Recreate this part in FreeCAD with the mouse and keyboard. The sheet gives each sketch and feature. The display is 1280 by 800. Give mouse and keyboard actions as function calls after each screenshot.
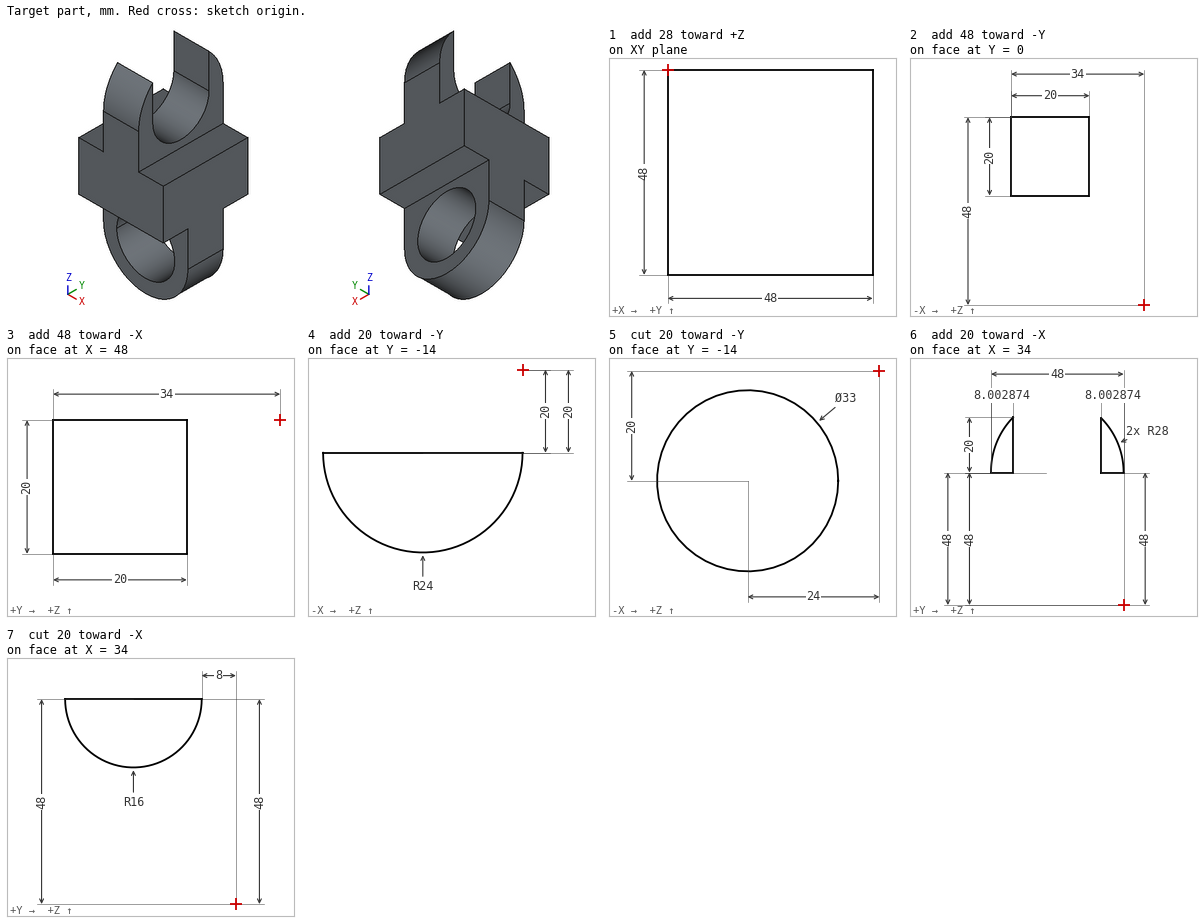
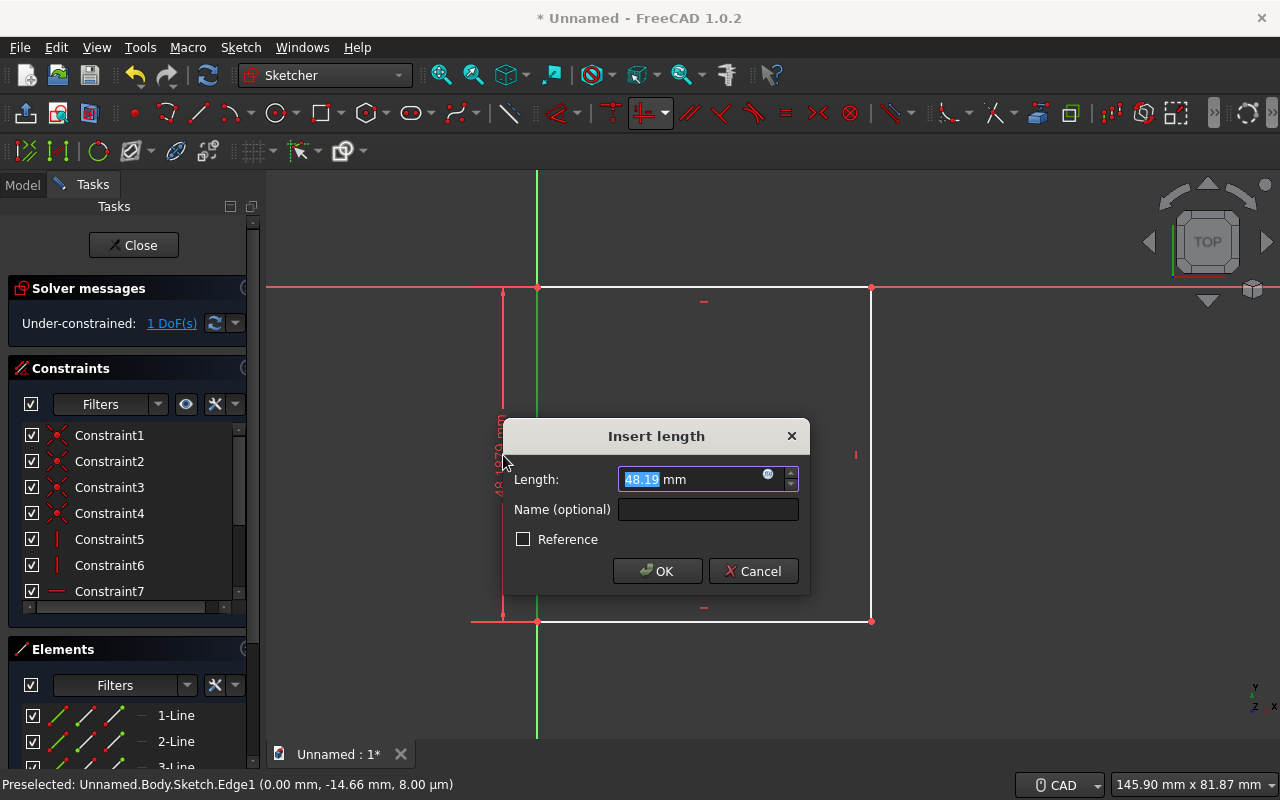
text(48)
key(Return)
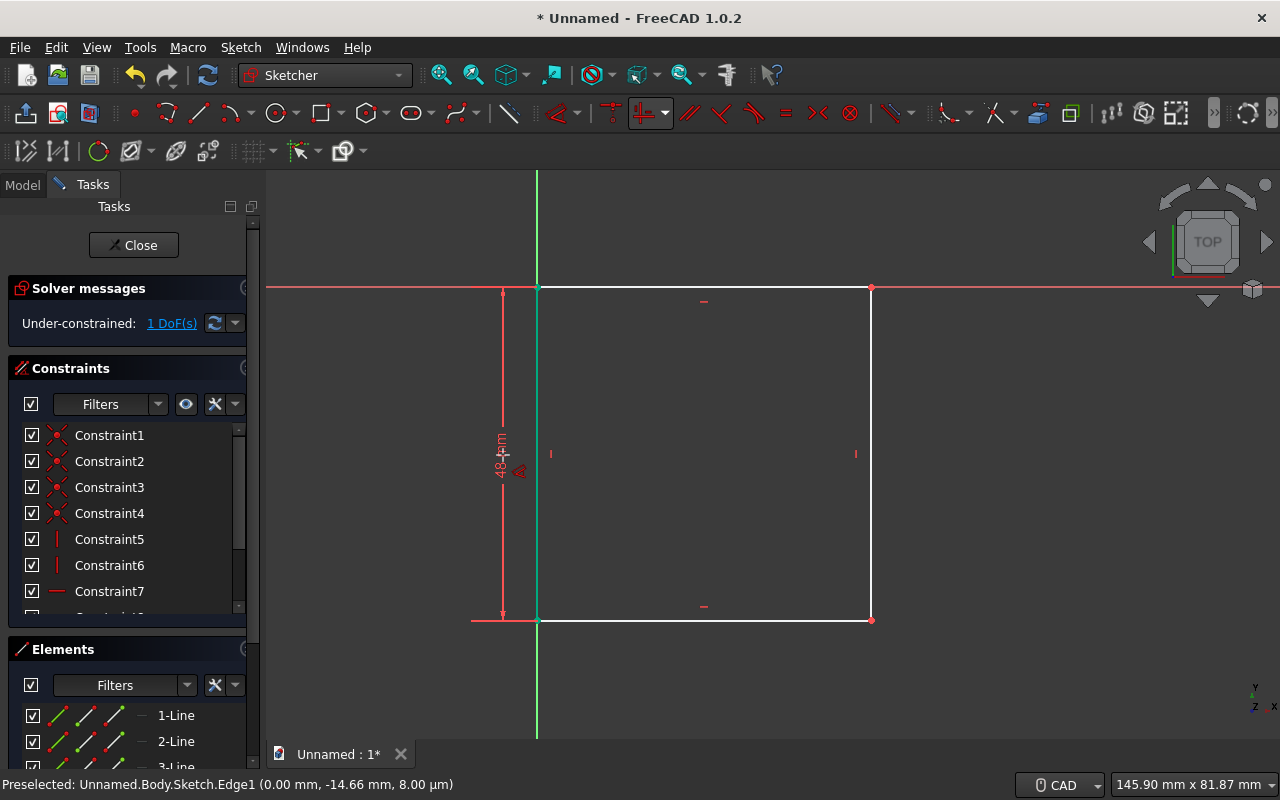
click(637, 621)
click(704, 655)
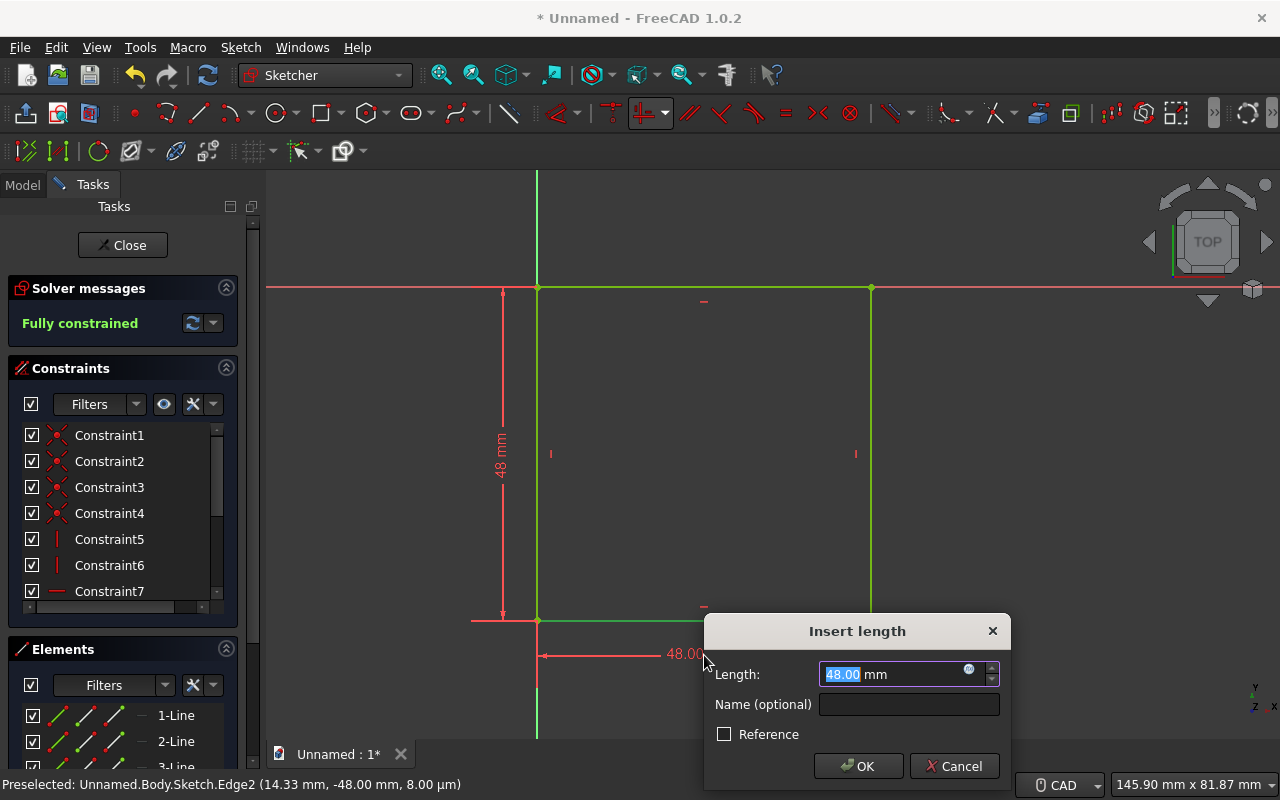
text(48)
key(Return)
key(Escape)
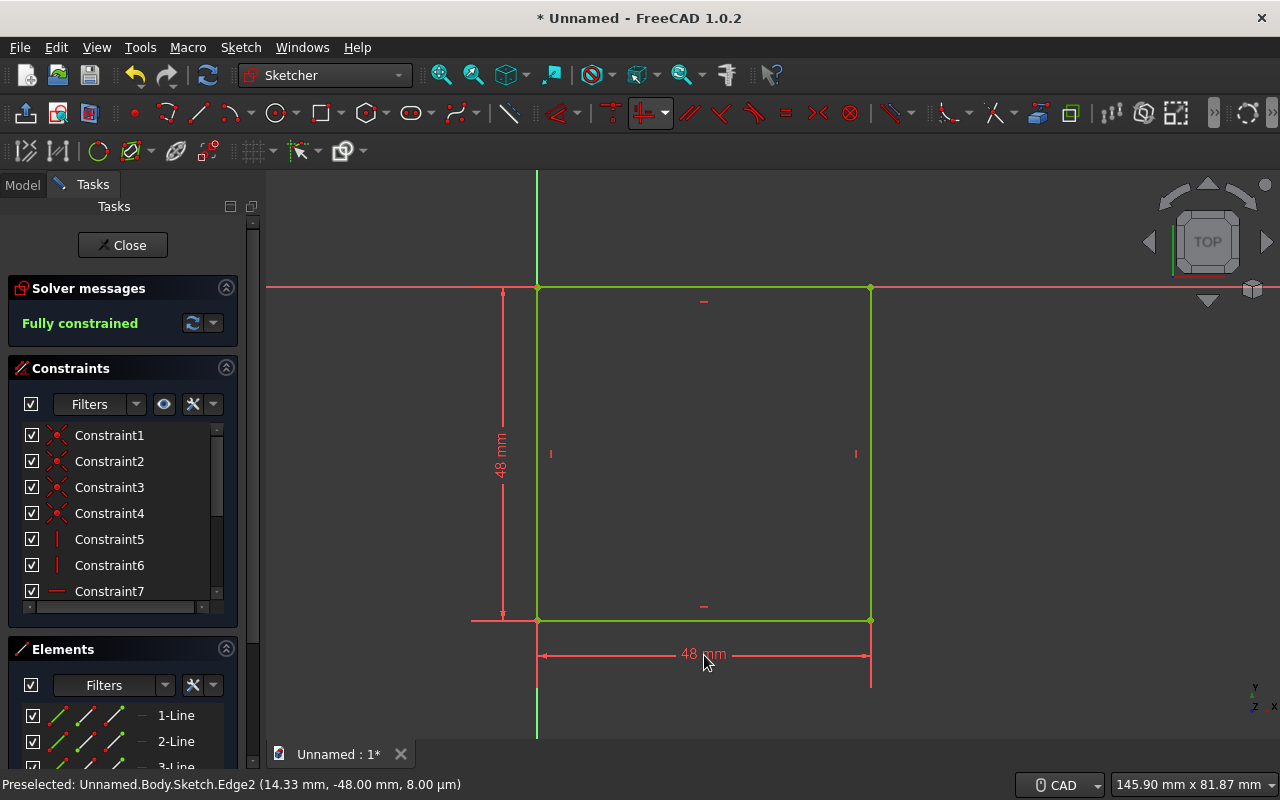
click(123, 245)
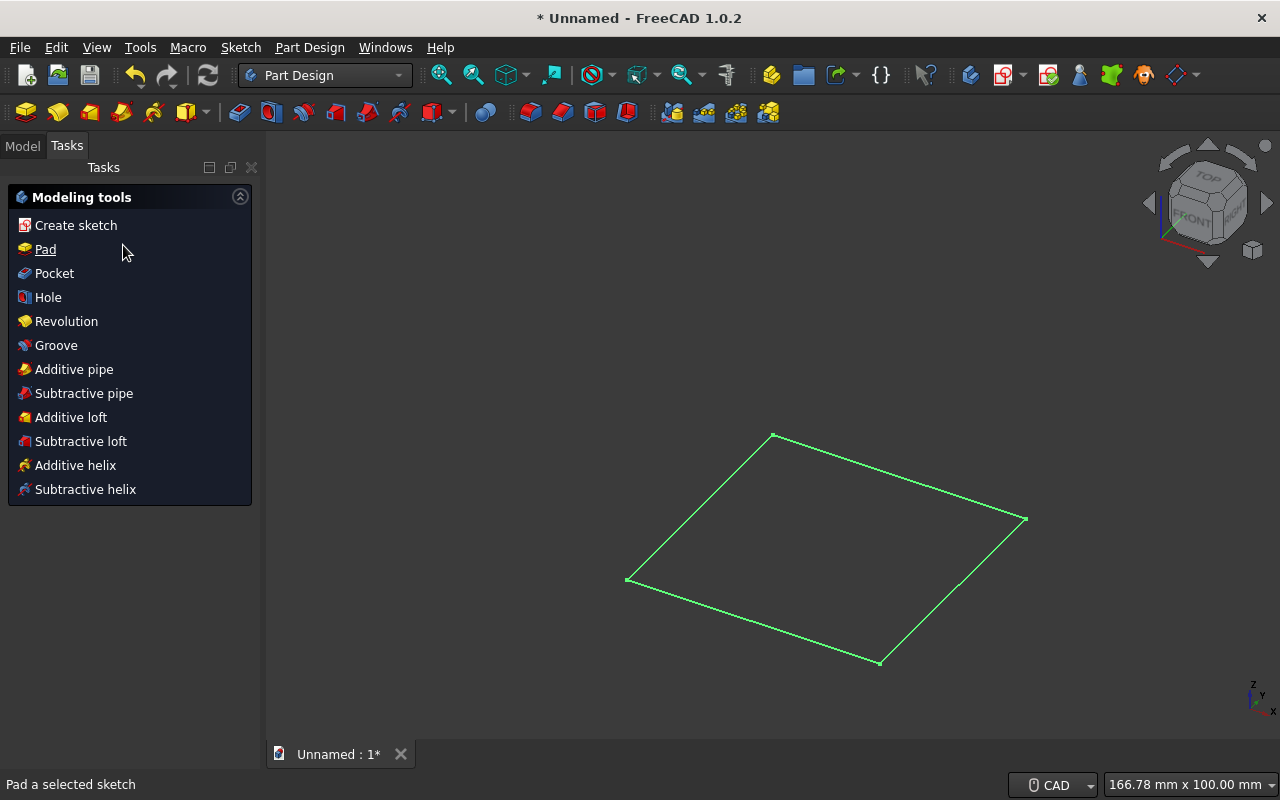
click(26, 112)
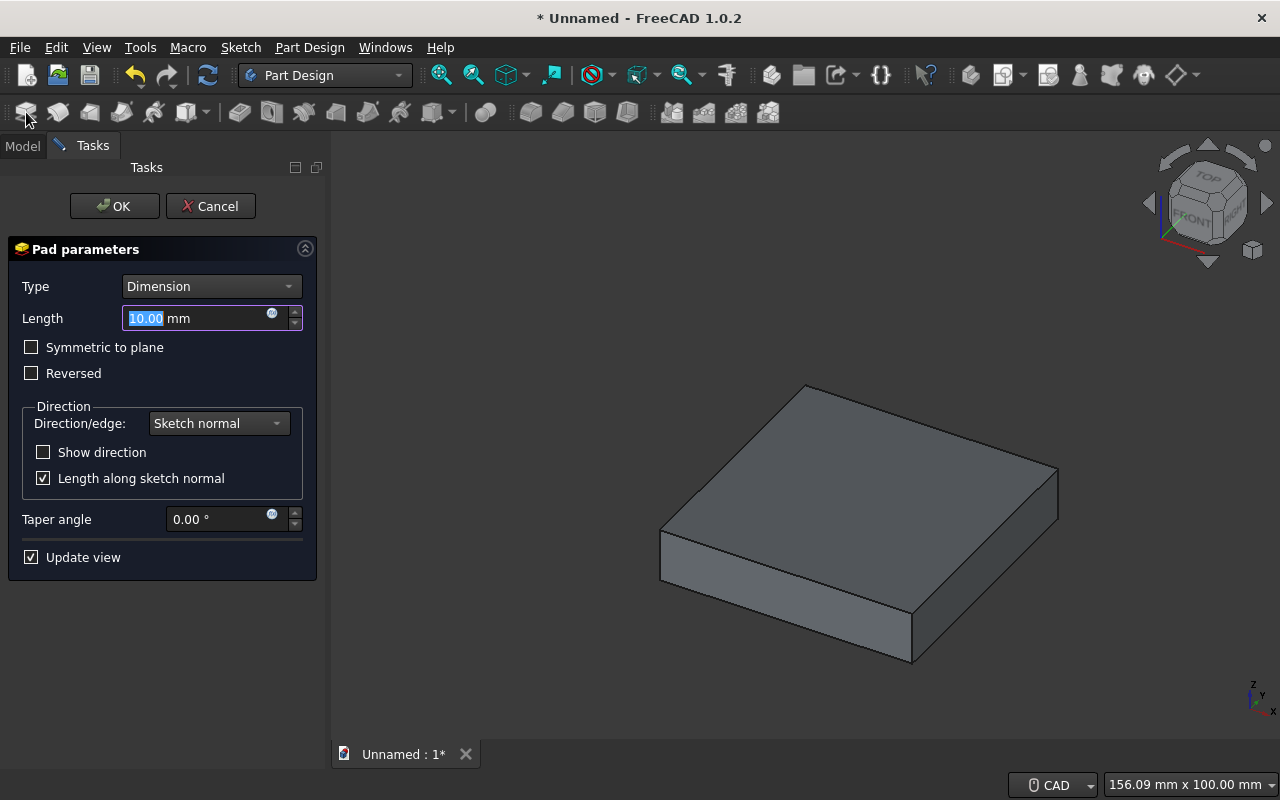
text(28)
key(Tab)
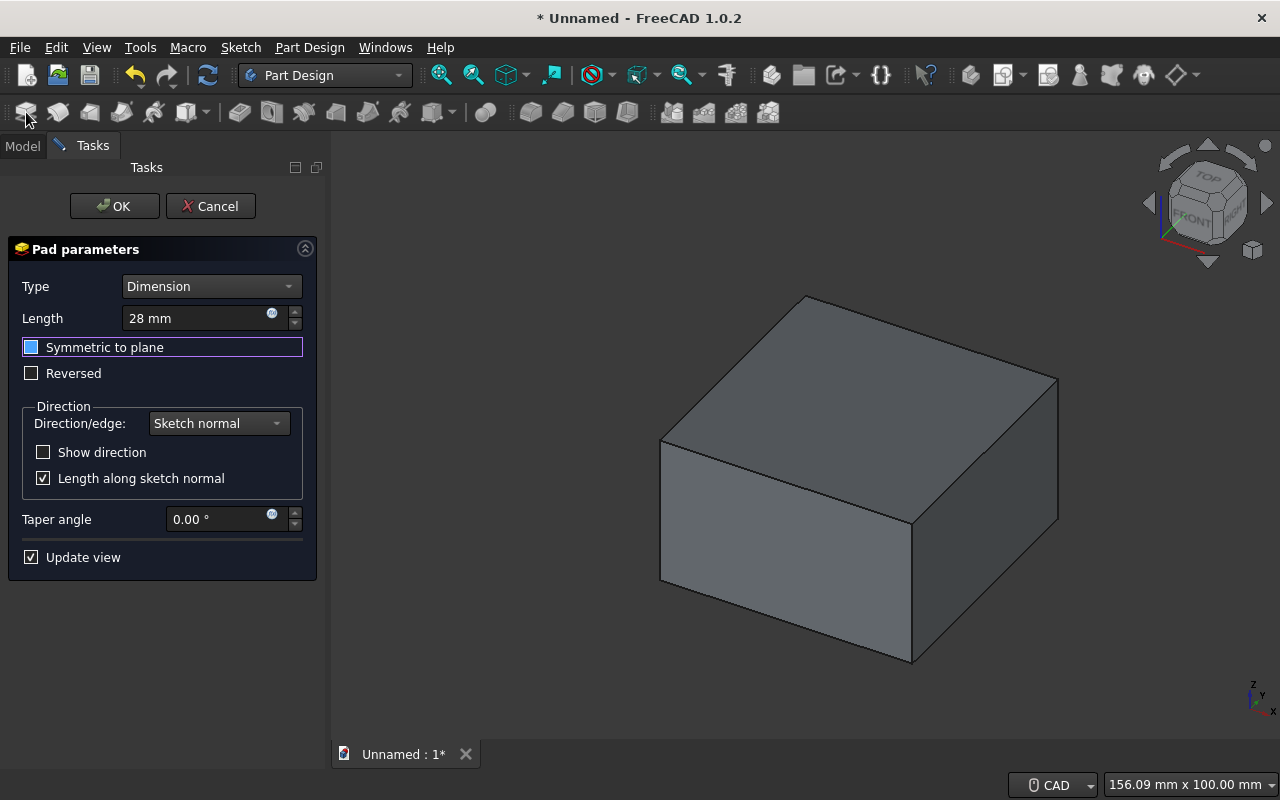
click(115, 206)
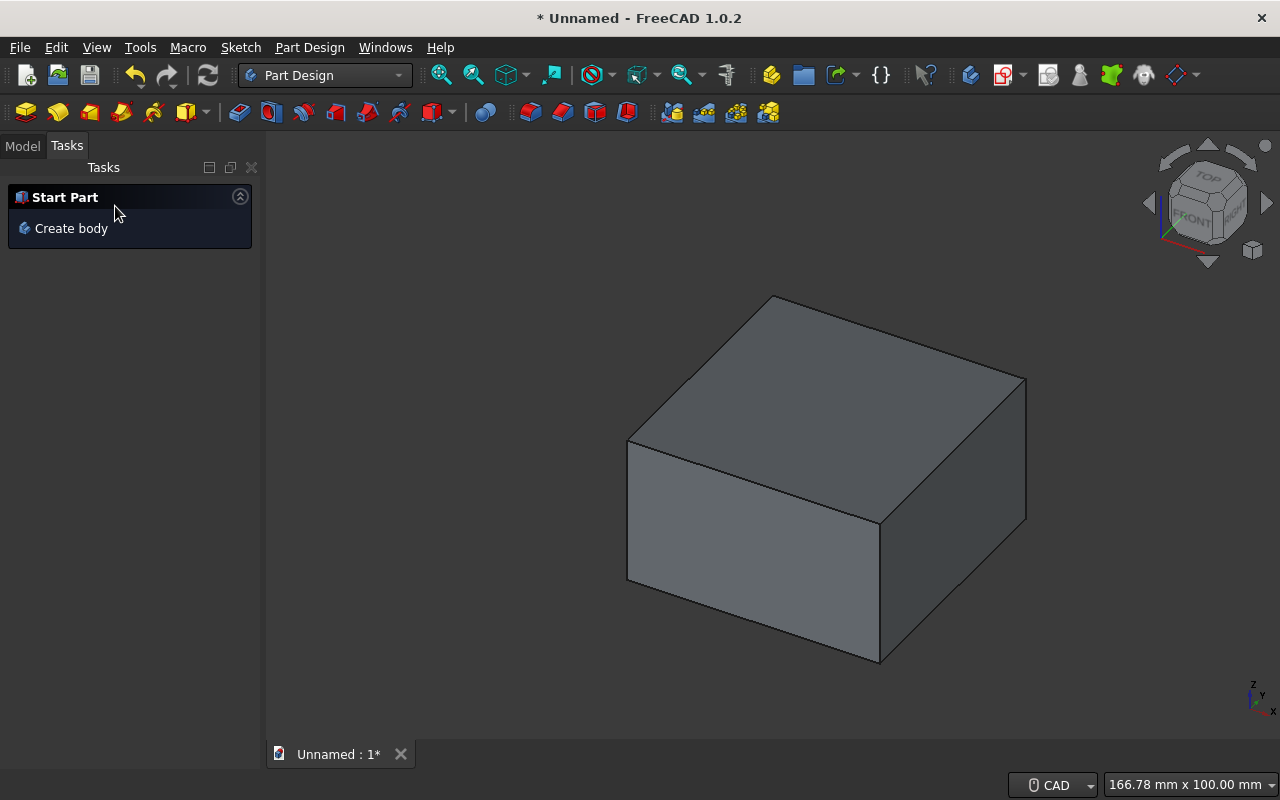
key(4)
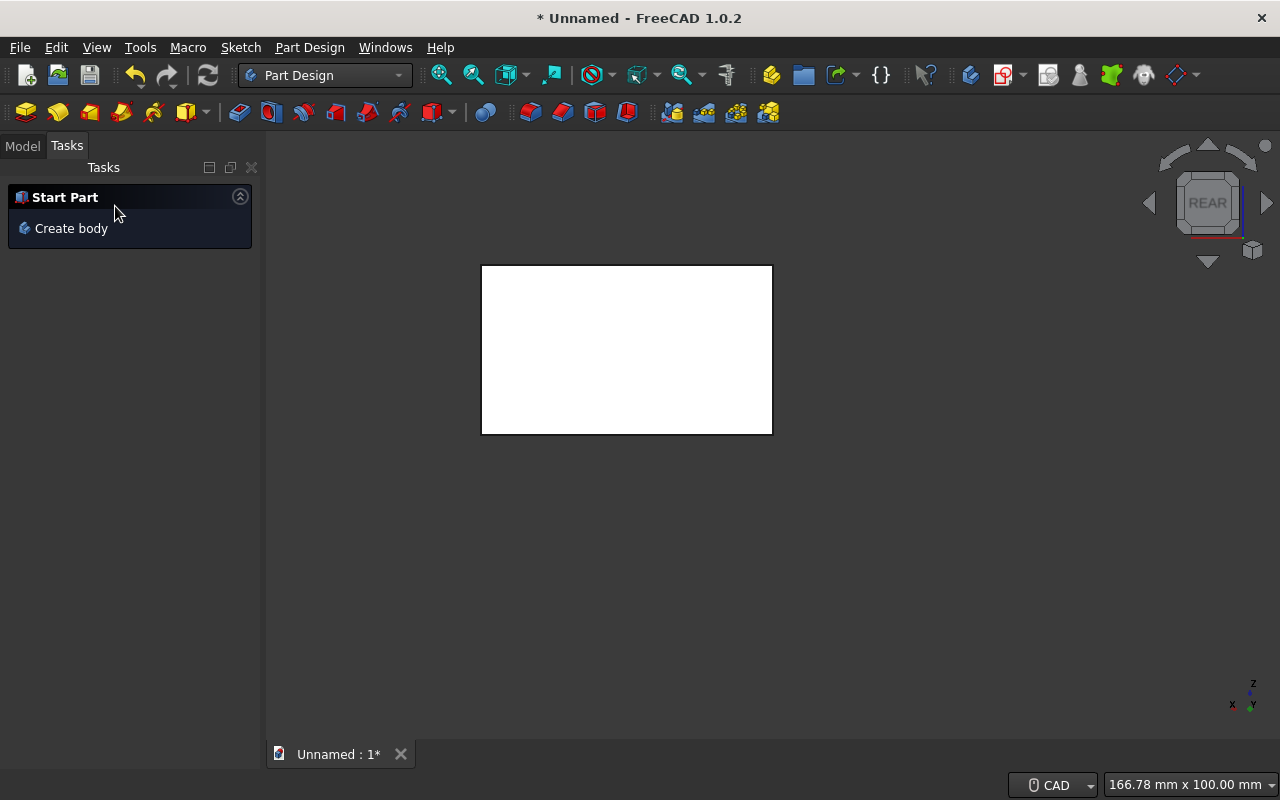
key(v)
key(f)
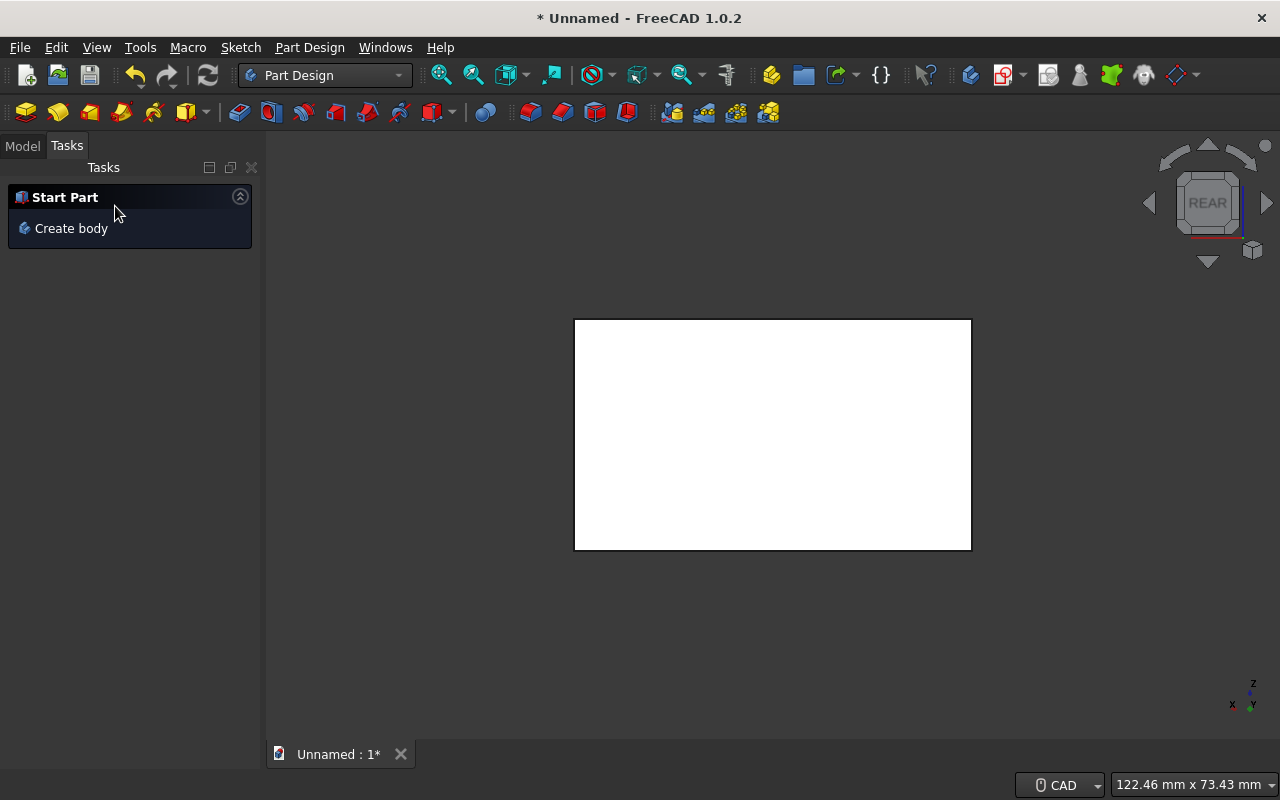
click(716, 434)